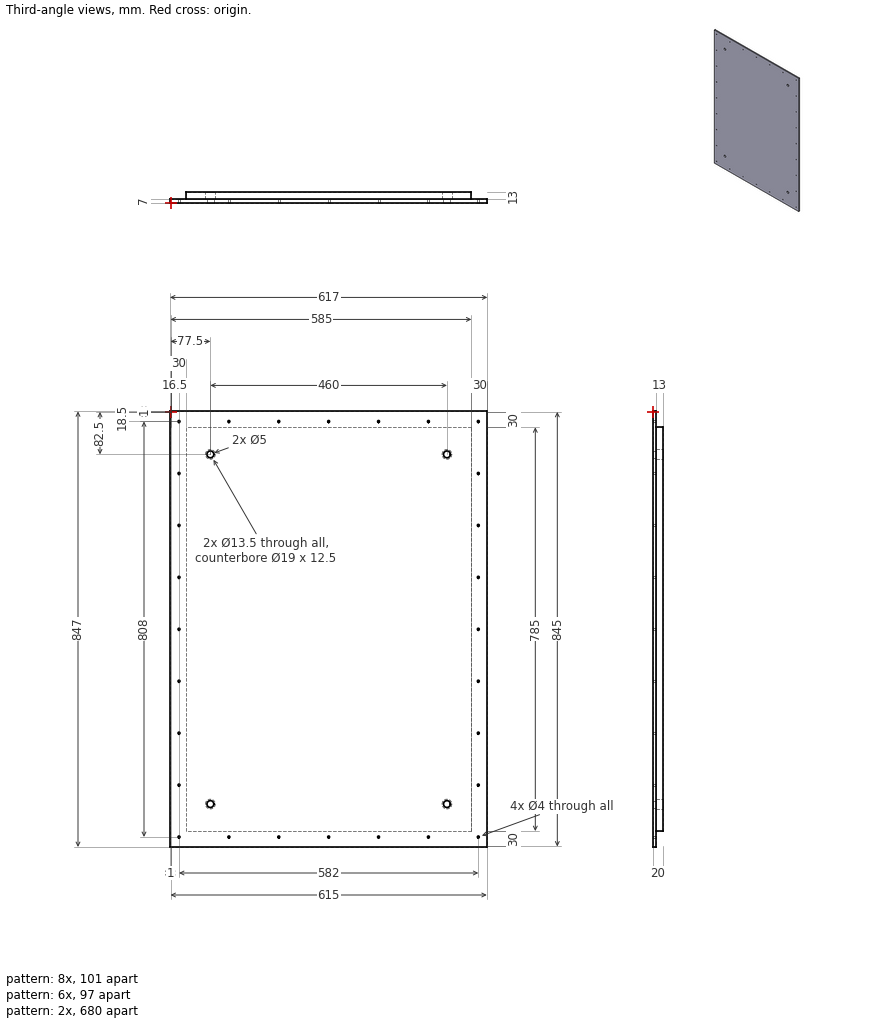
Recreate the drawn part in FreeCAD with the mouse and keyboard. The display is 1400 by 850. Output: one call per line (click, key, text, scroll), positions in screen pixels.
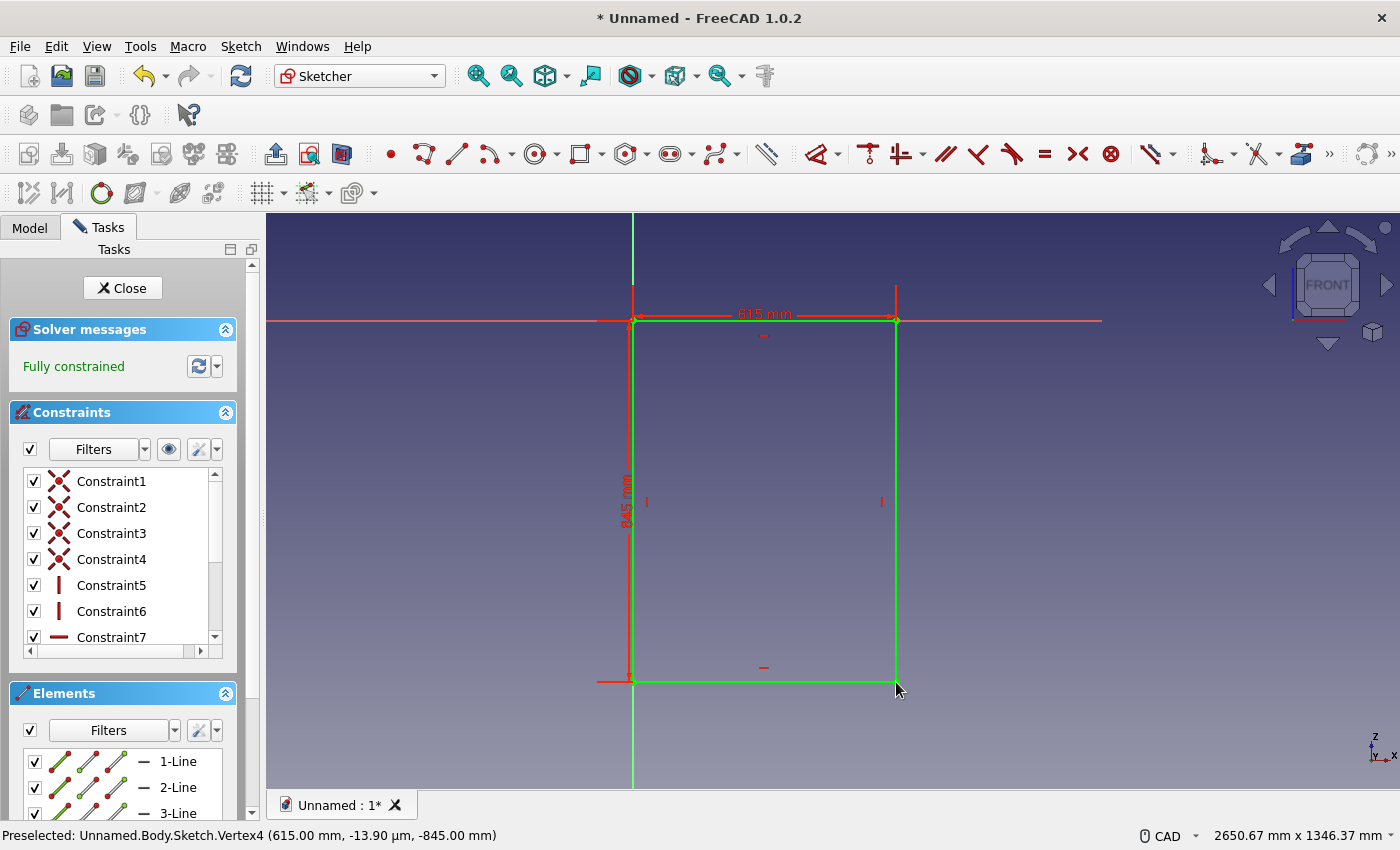
click(123, 288)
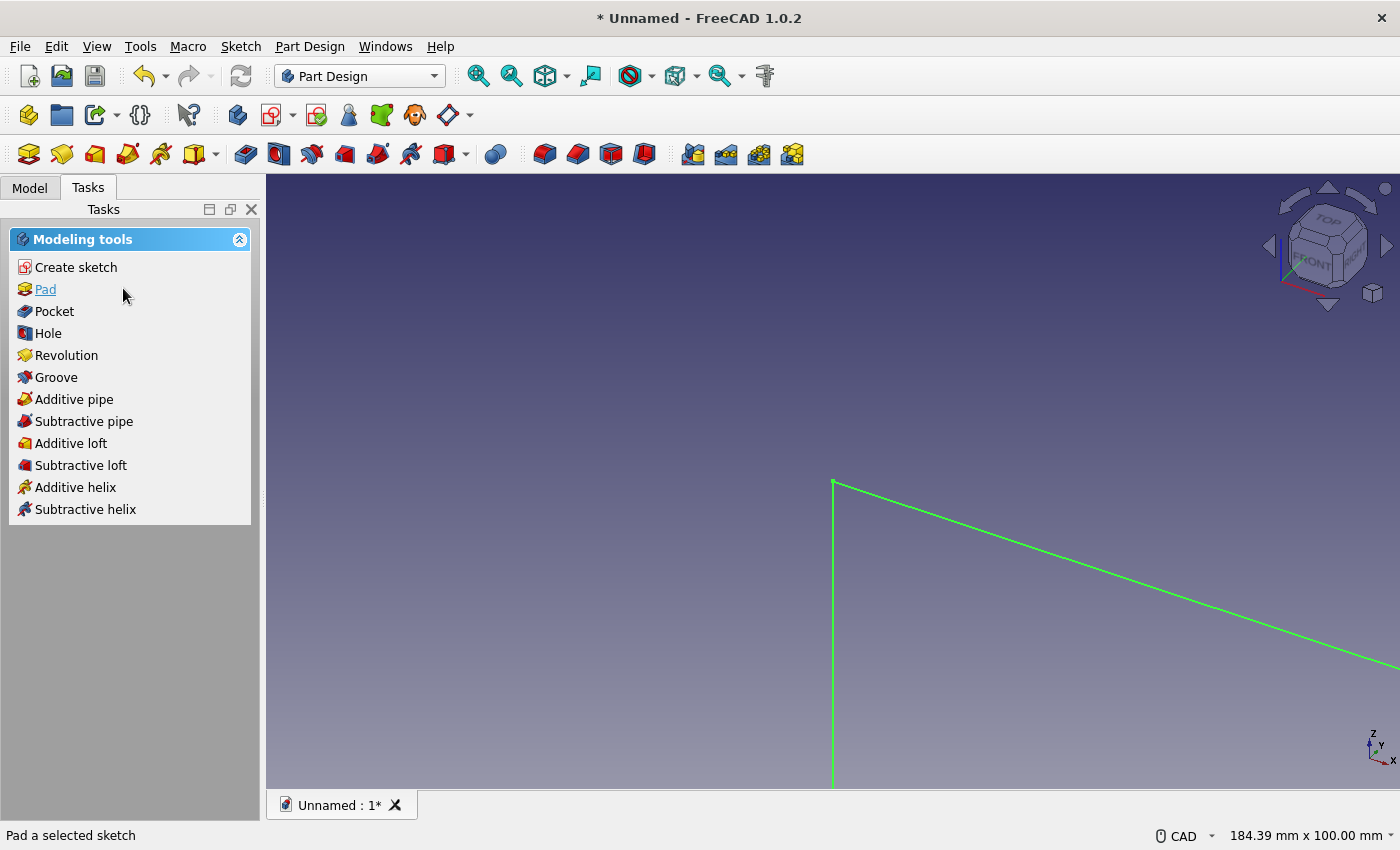
click(29, 154)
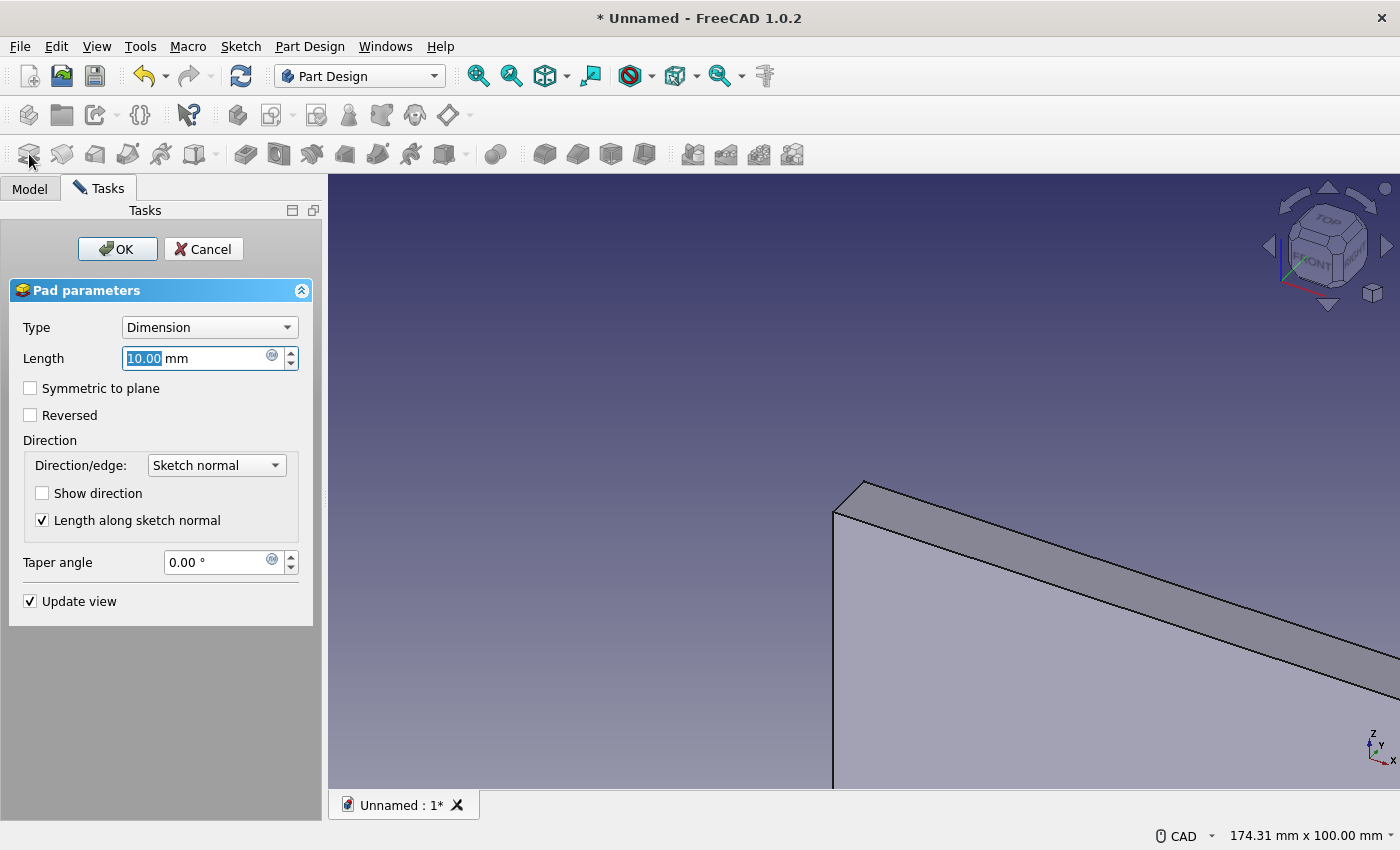
text(20)
key(Tab)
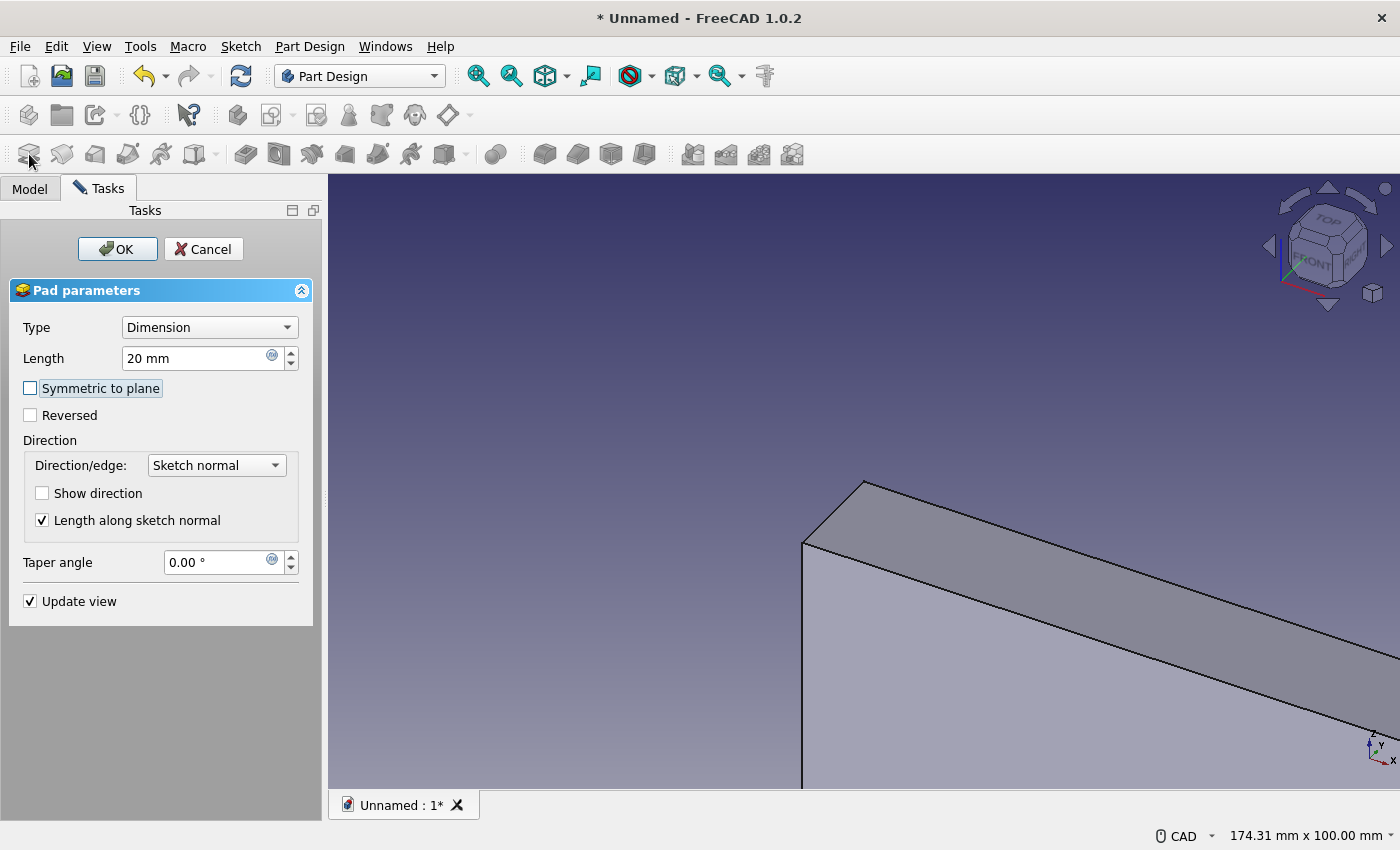
click(31, 415)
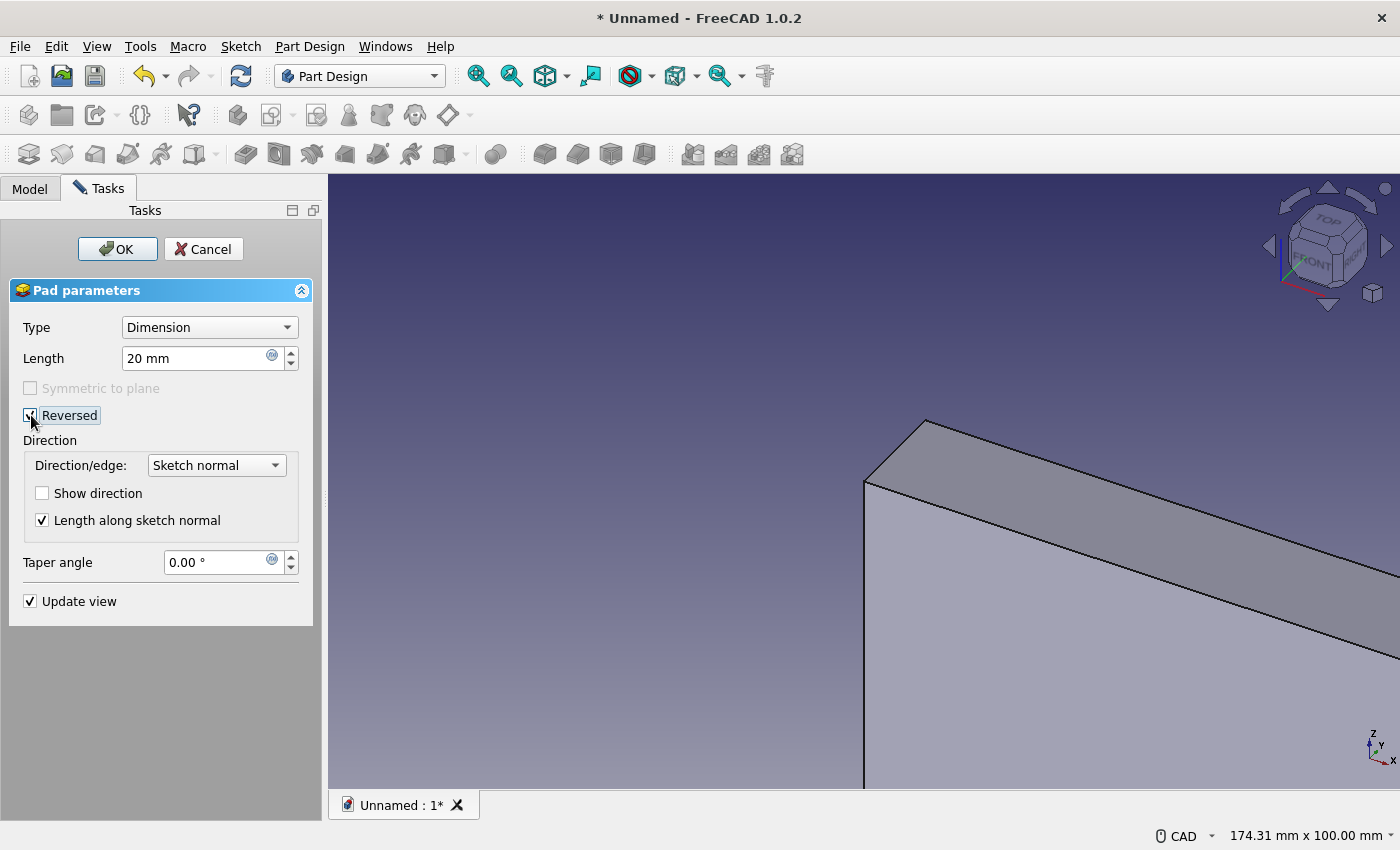
click(118, 249)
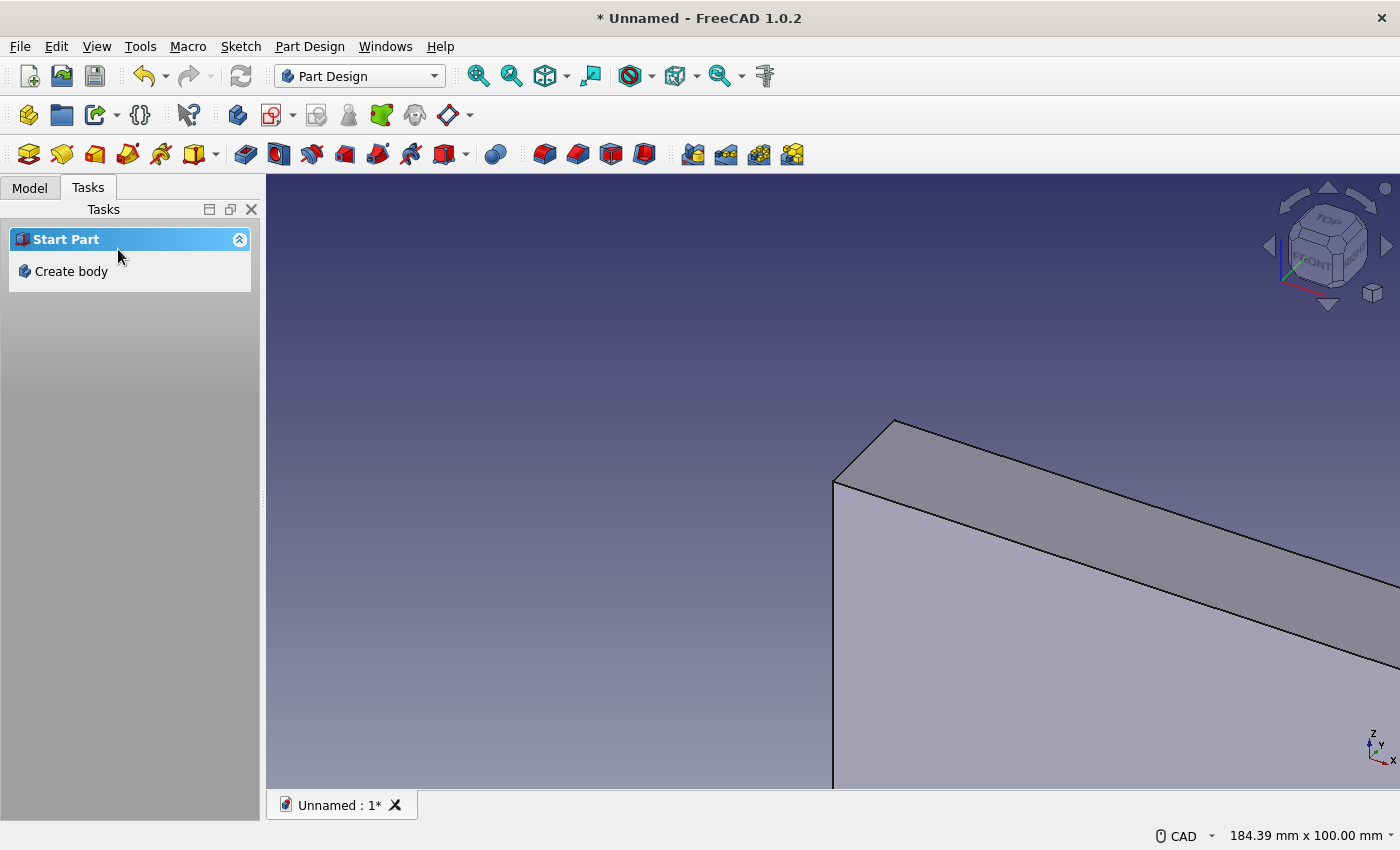
click(479, 76)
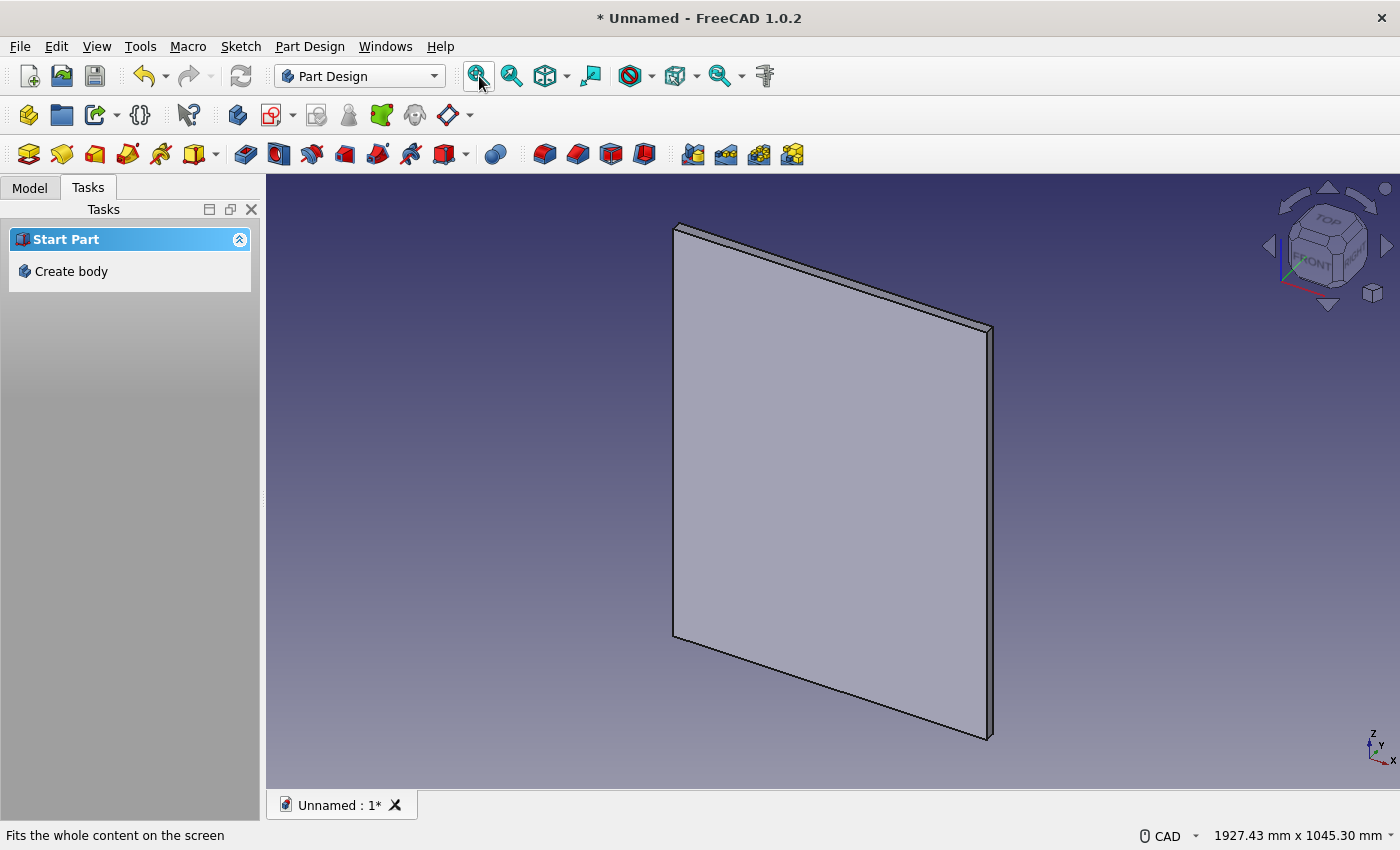
key(4)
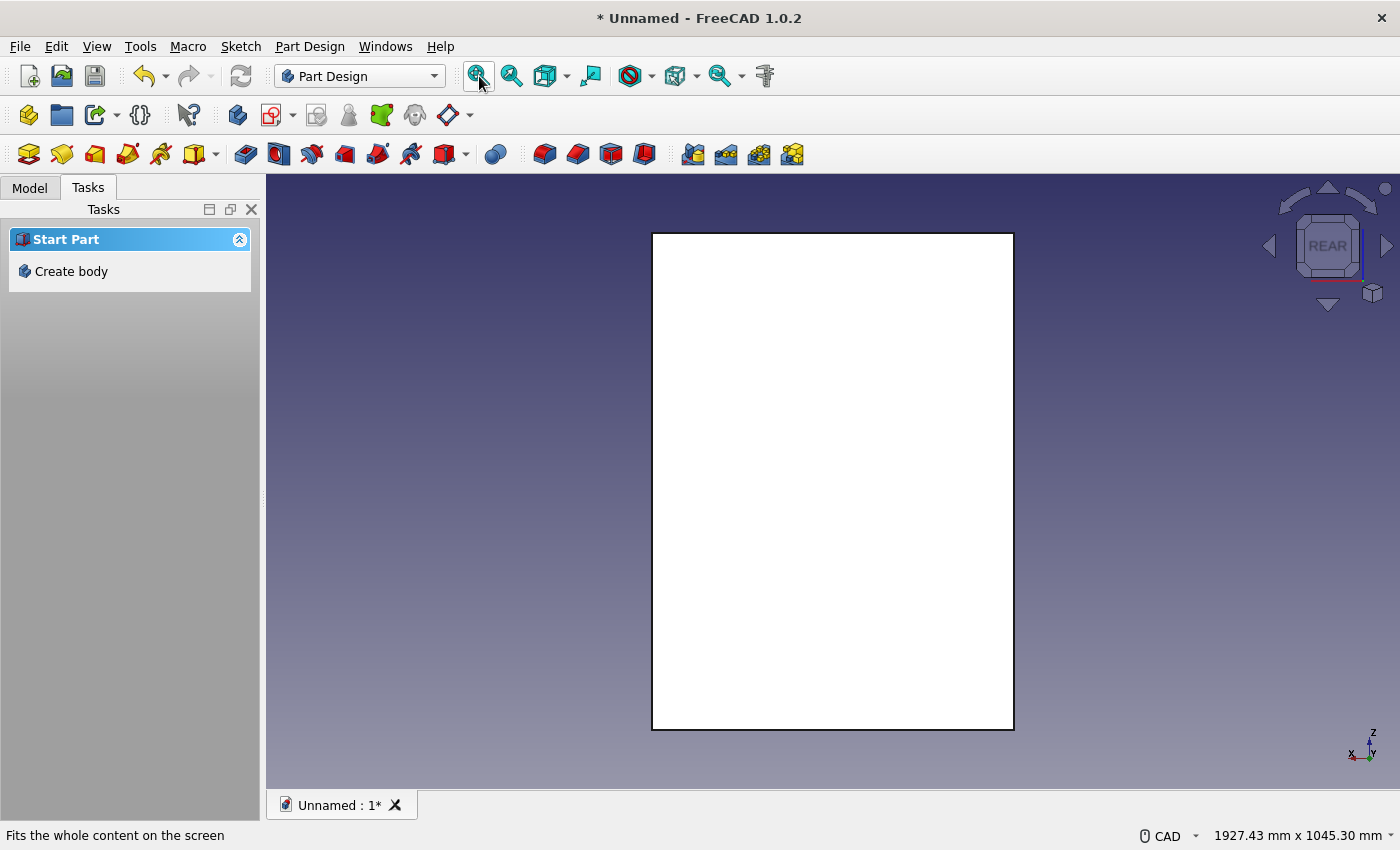
click(833, 480)